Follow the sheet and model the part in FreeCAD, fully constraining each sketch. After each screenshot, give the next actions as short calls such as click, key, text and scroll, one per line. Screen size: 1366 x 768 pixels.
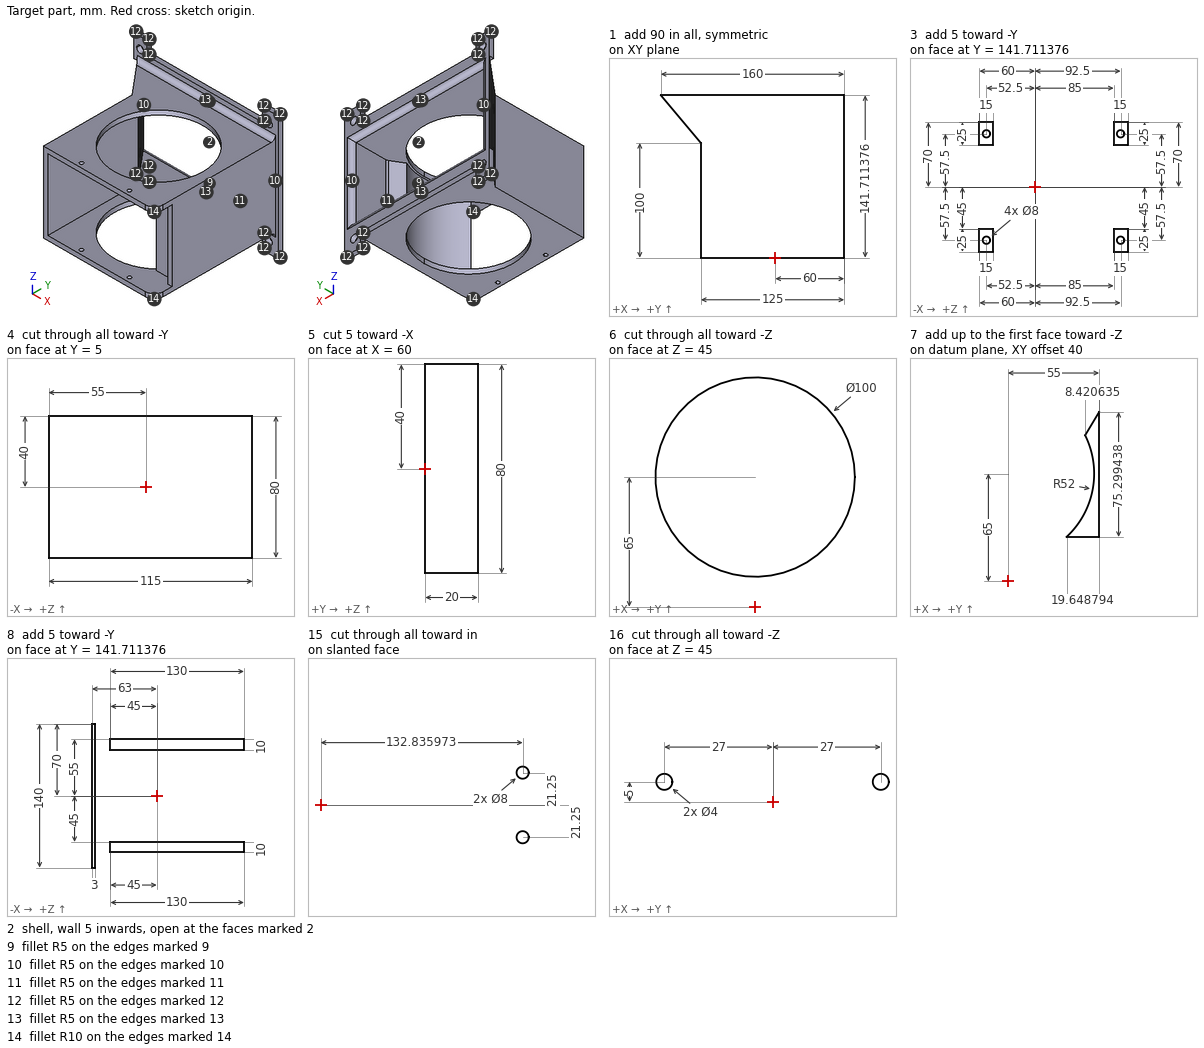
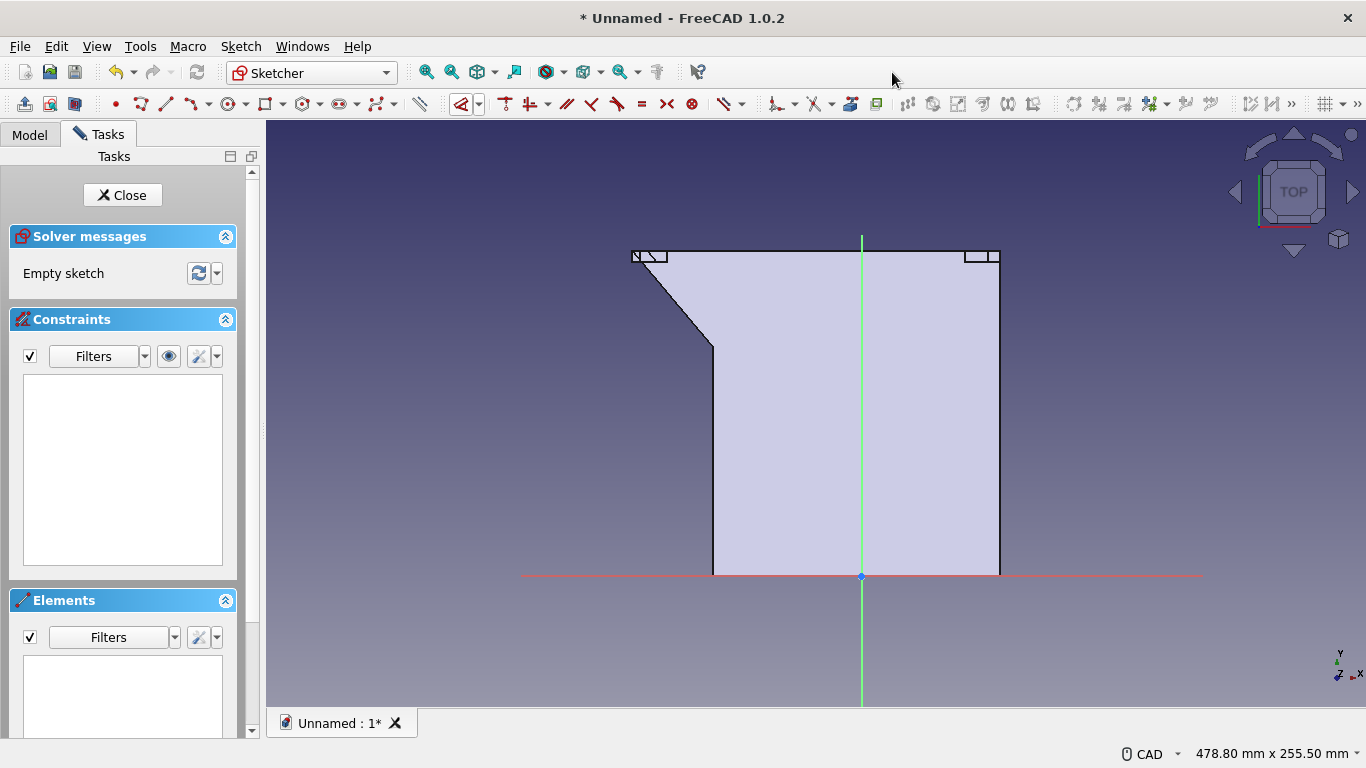
scroll(1095, 507, up, 2)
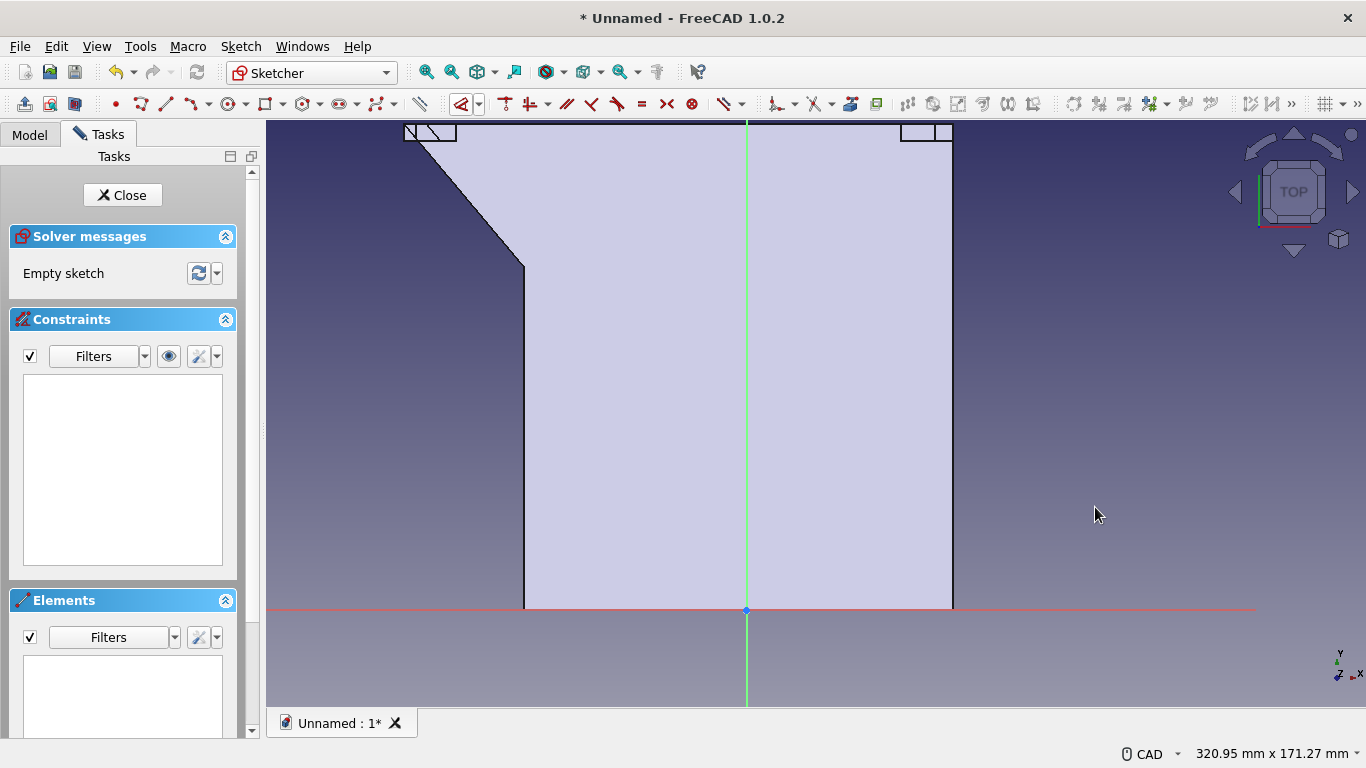
key(g)
key(c)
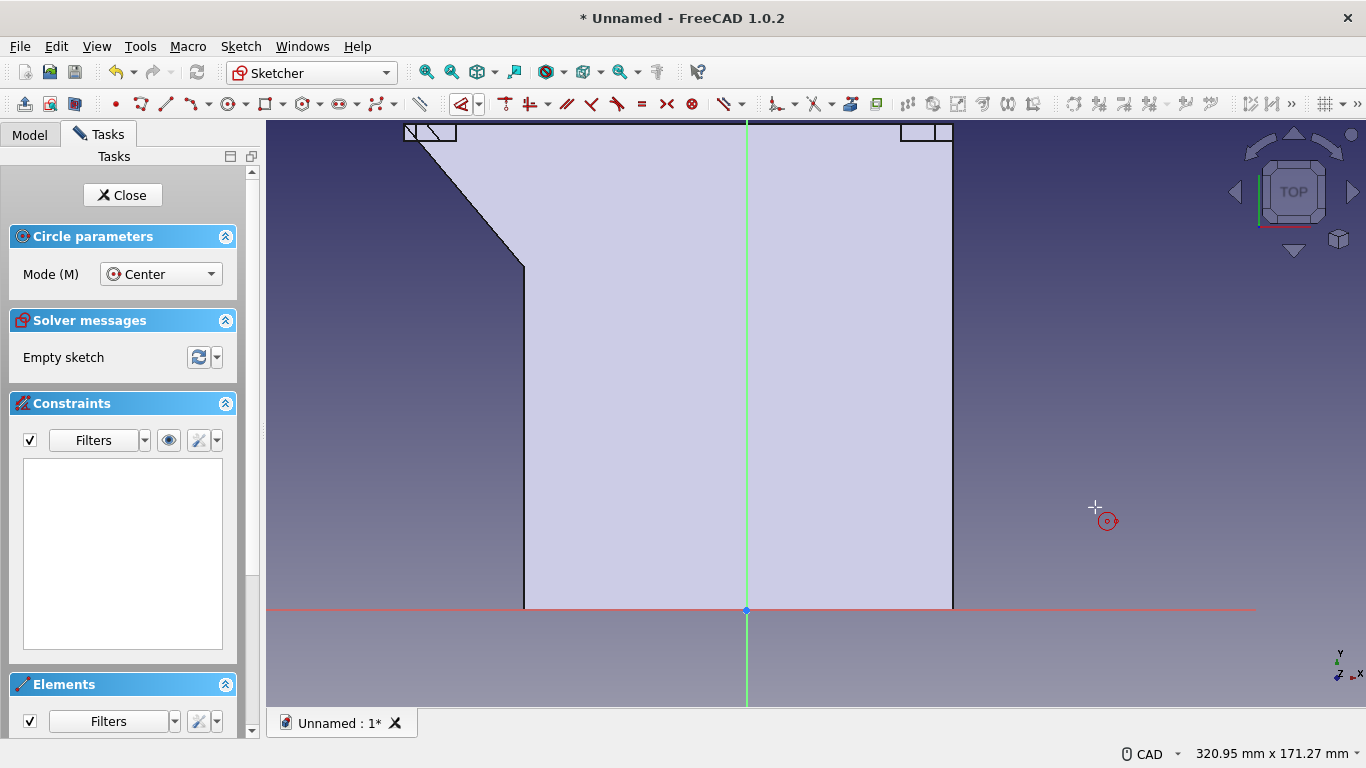
click(747, 387)
move(868, 266)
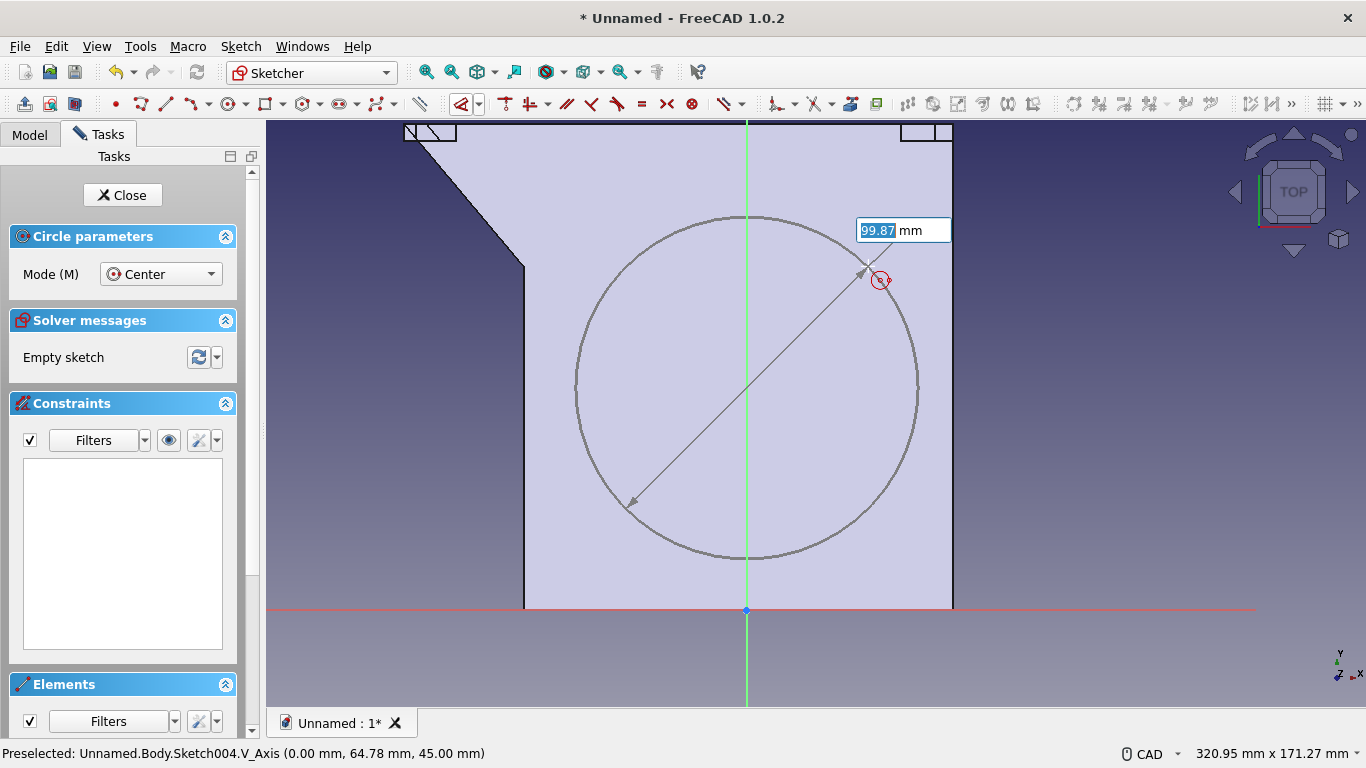
text(100)
key(Return)
key(Escape)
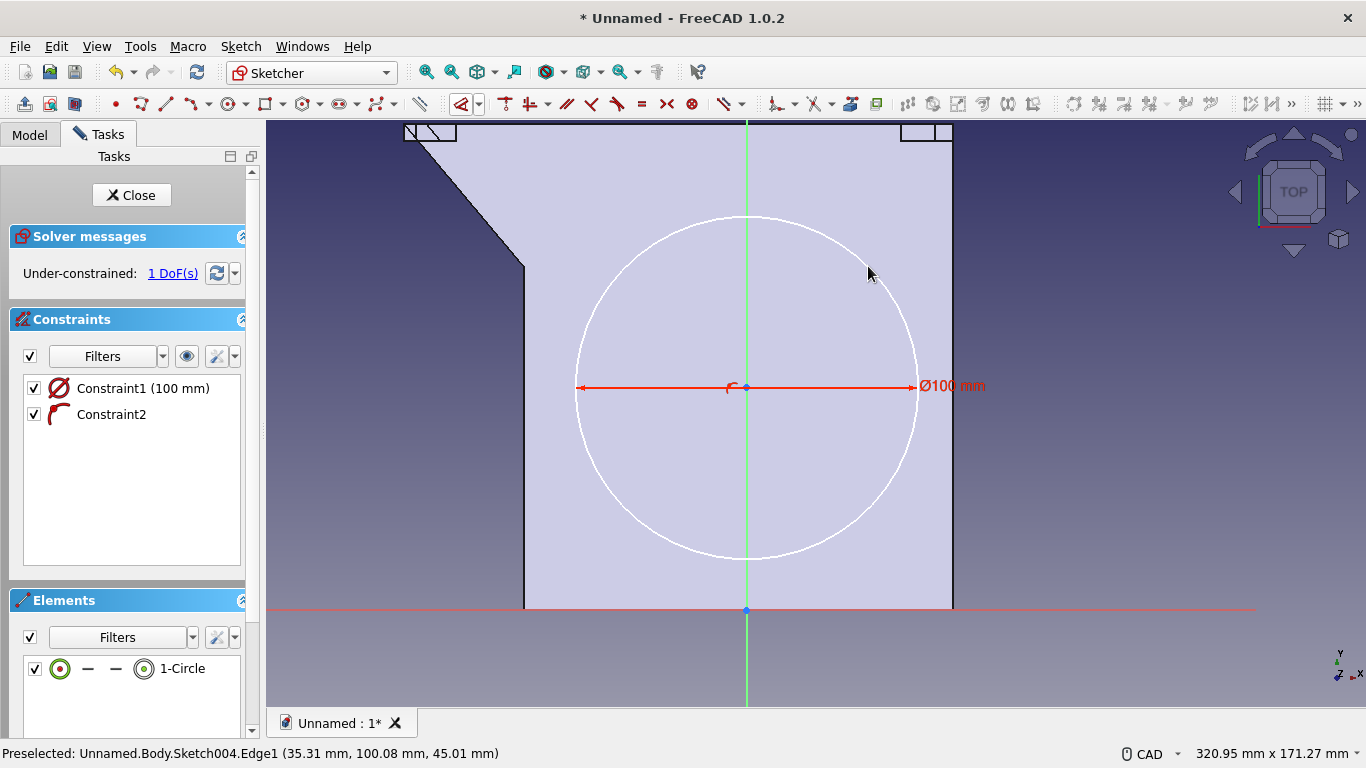
click(747, 388)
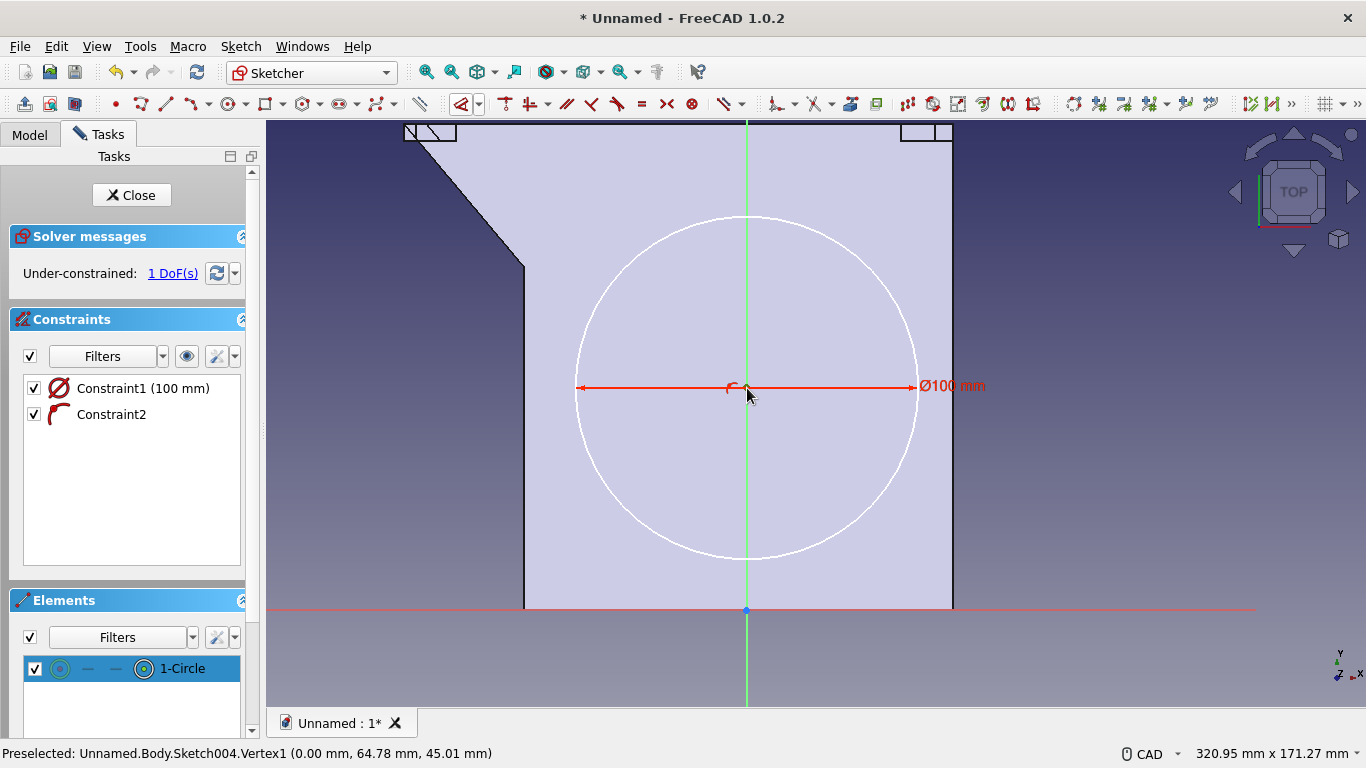
key(i)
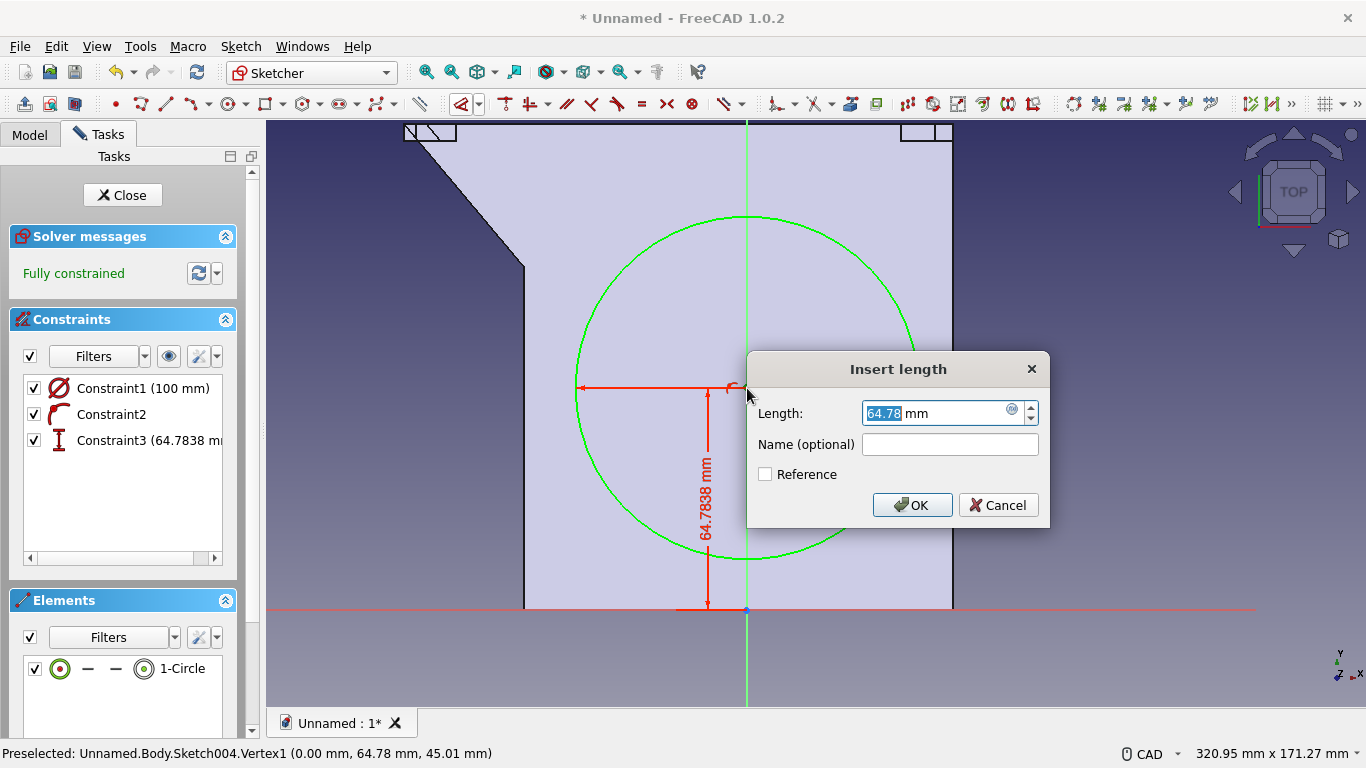
text(65)
key(Return)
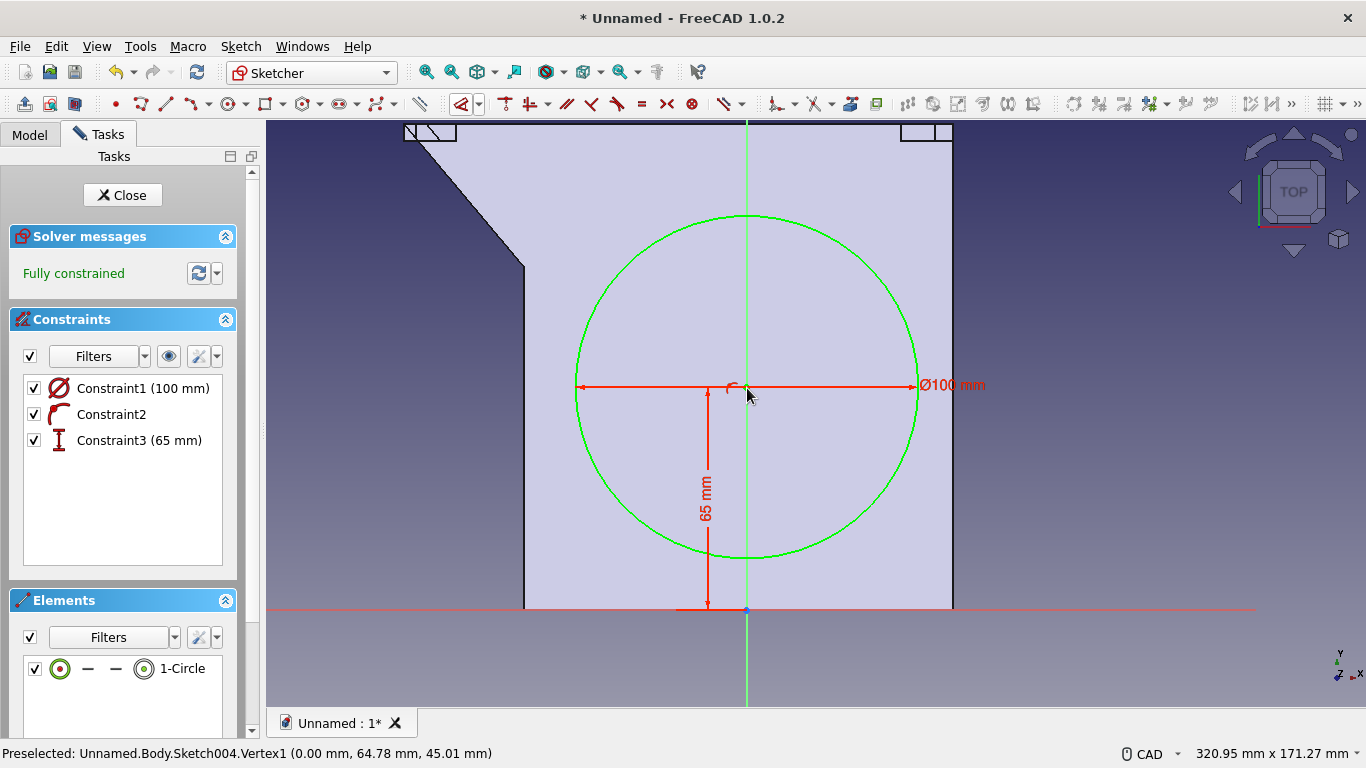
click(123, 195)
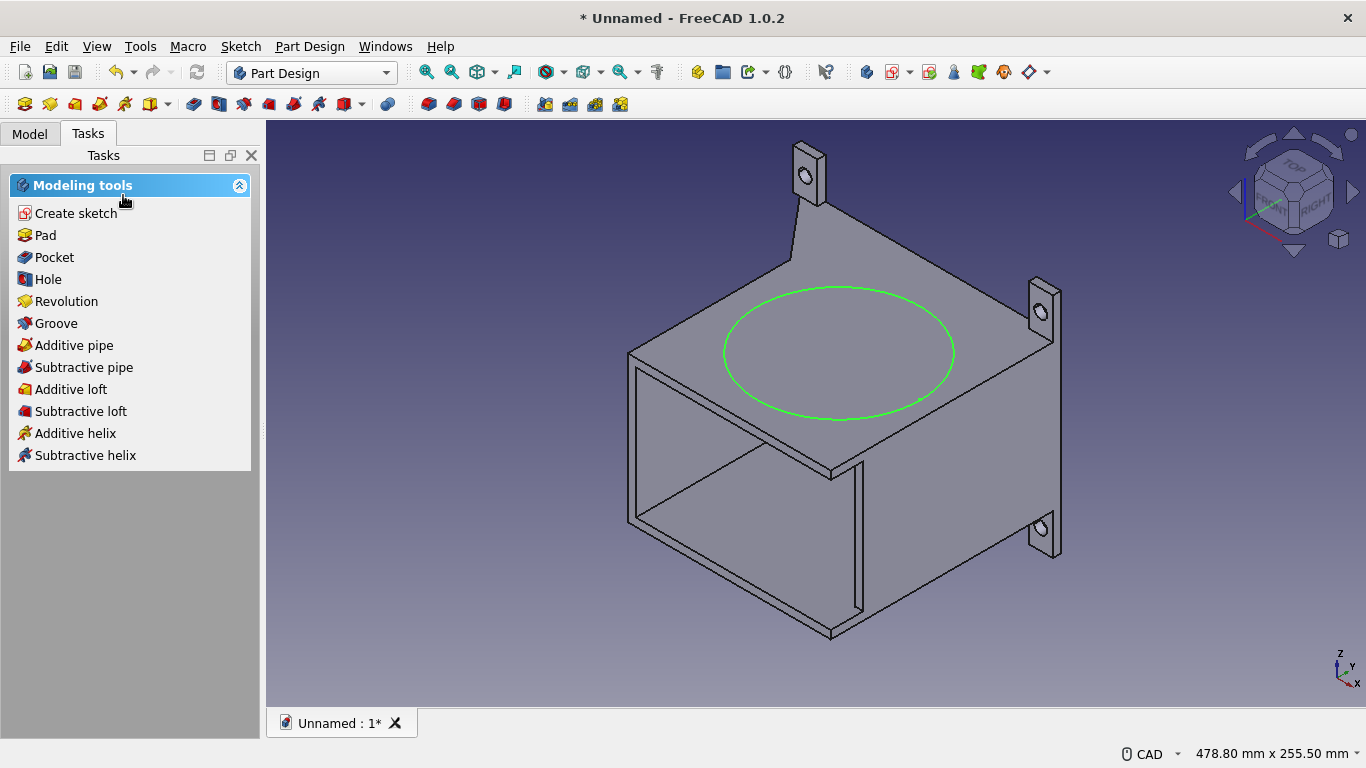
click(194, 104)